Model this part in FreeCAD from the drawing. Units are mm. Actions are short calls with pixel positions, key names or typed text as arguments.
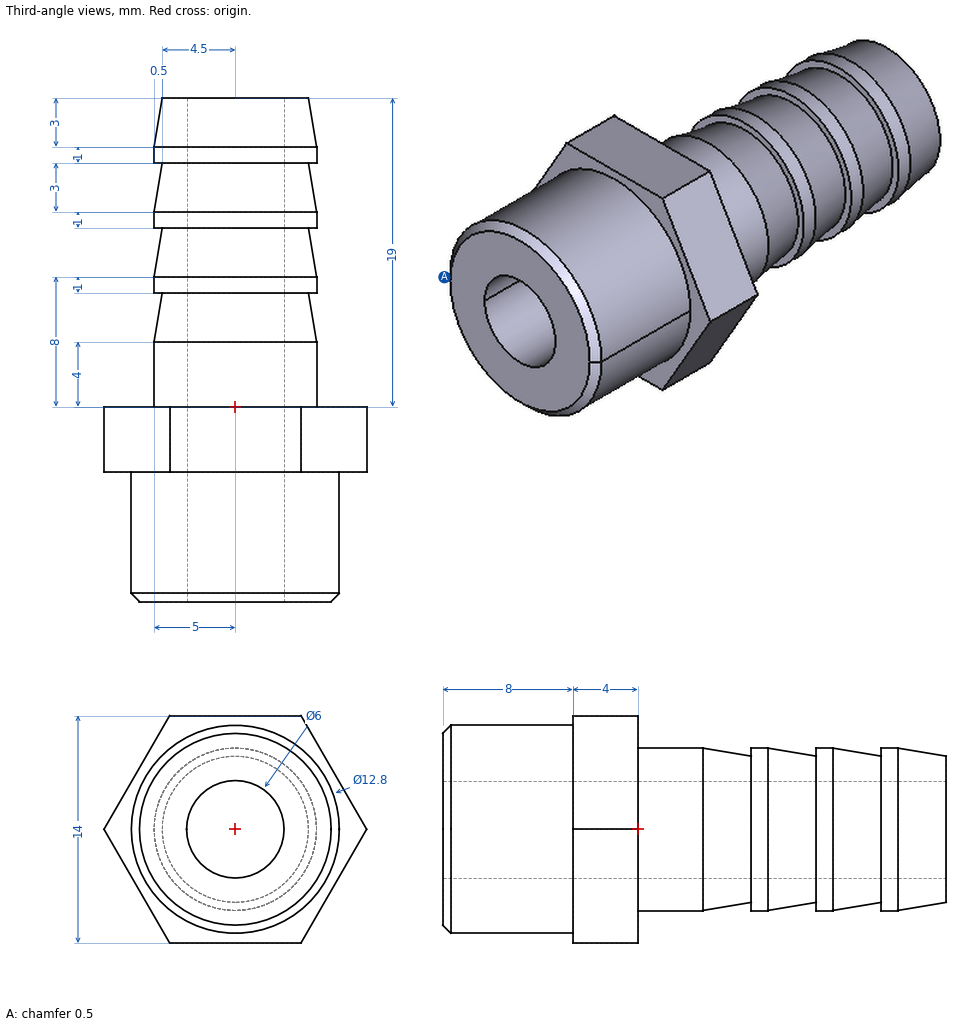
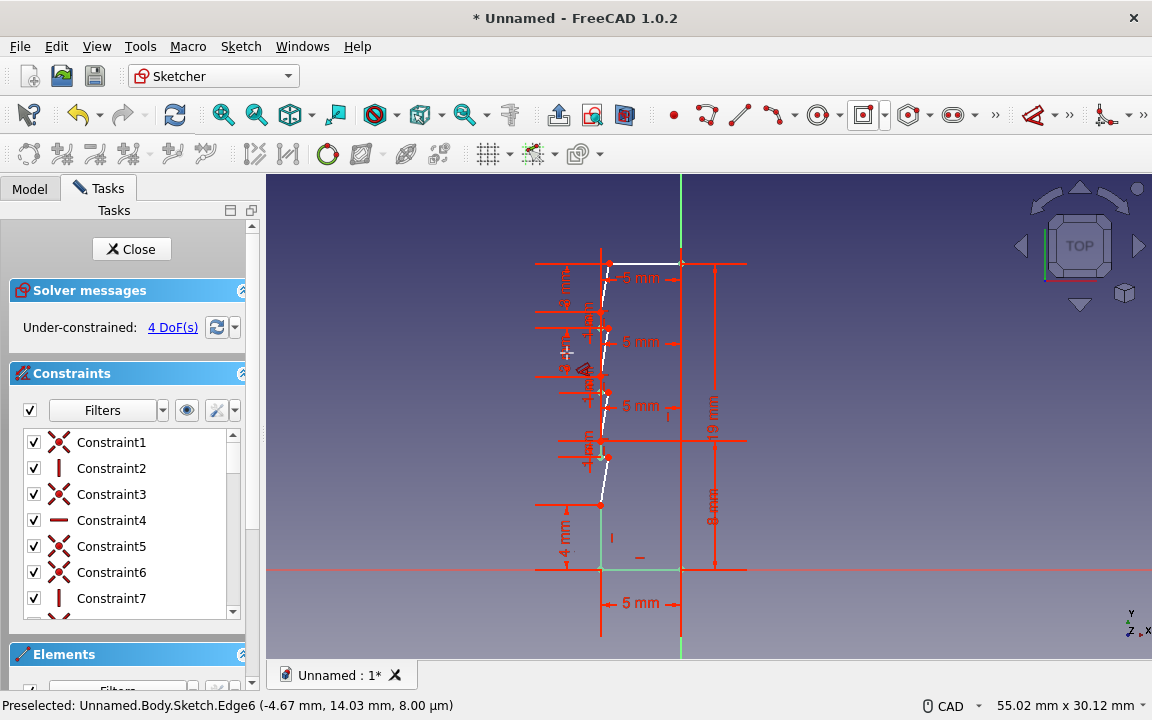
click(659, 264)
click(645, 230)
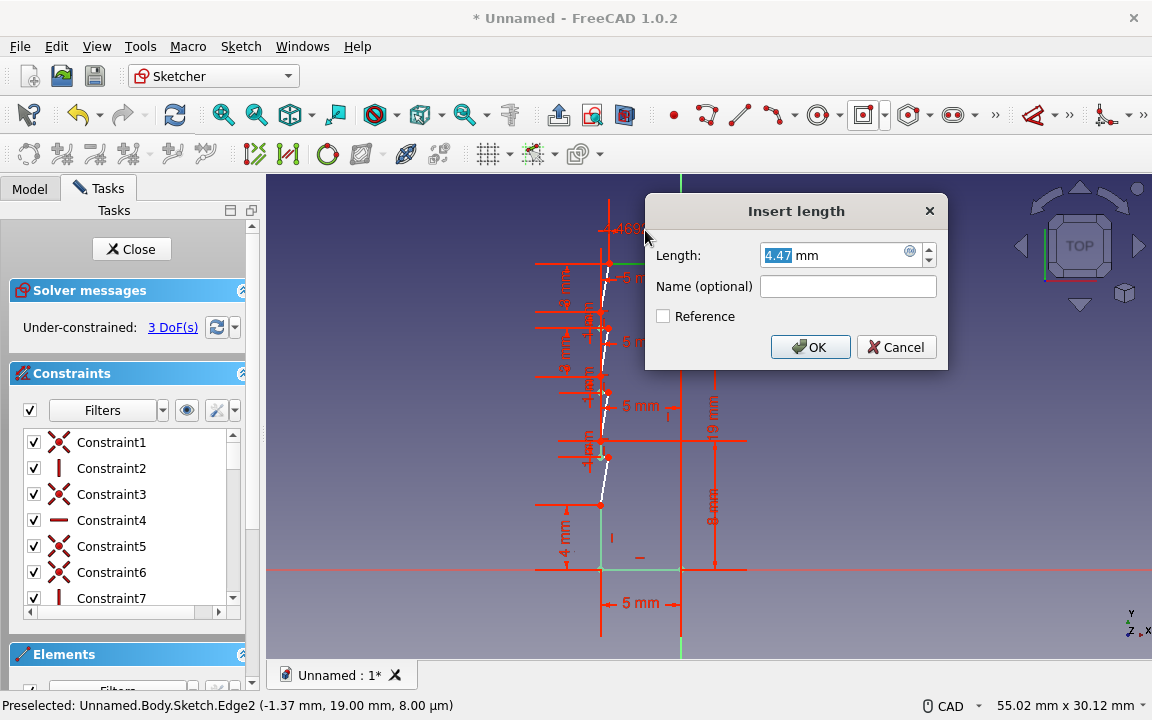
text(4.5)
key(Return)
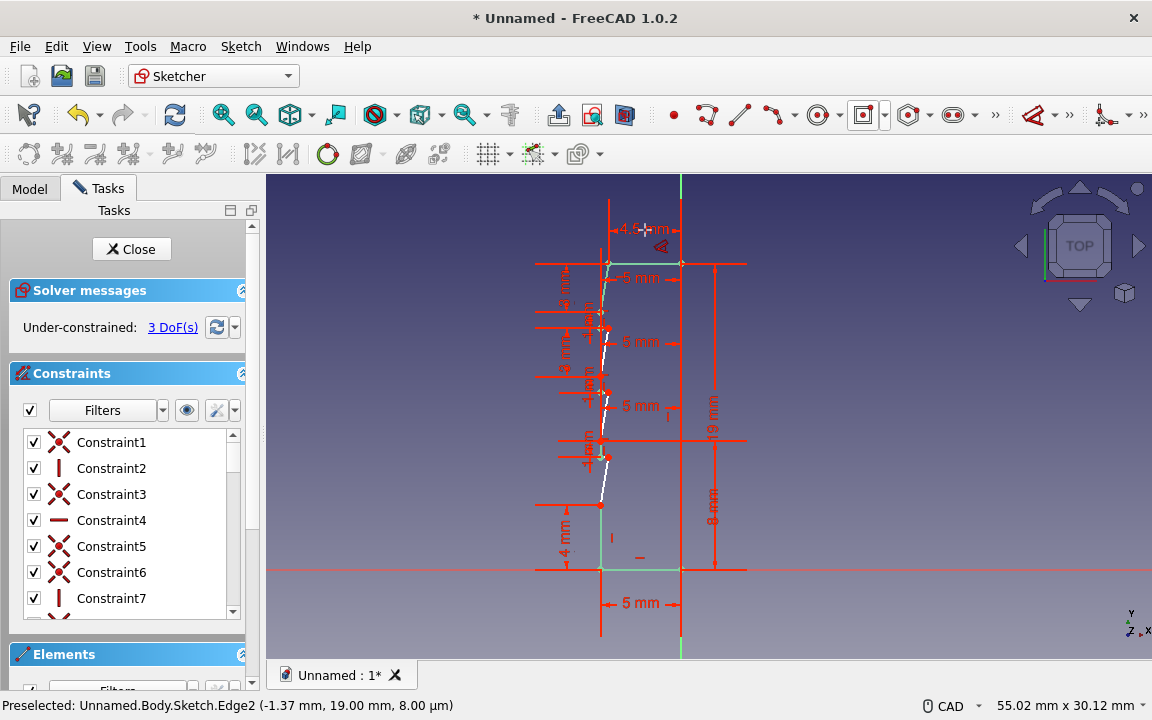
scroll(604, 328, up, 8)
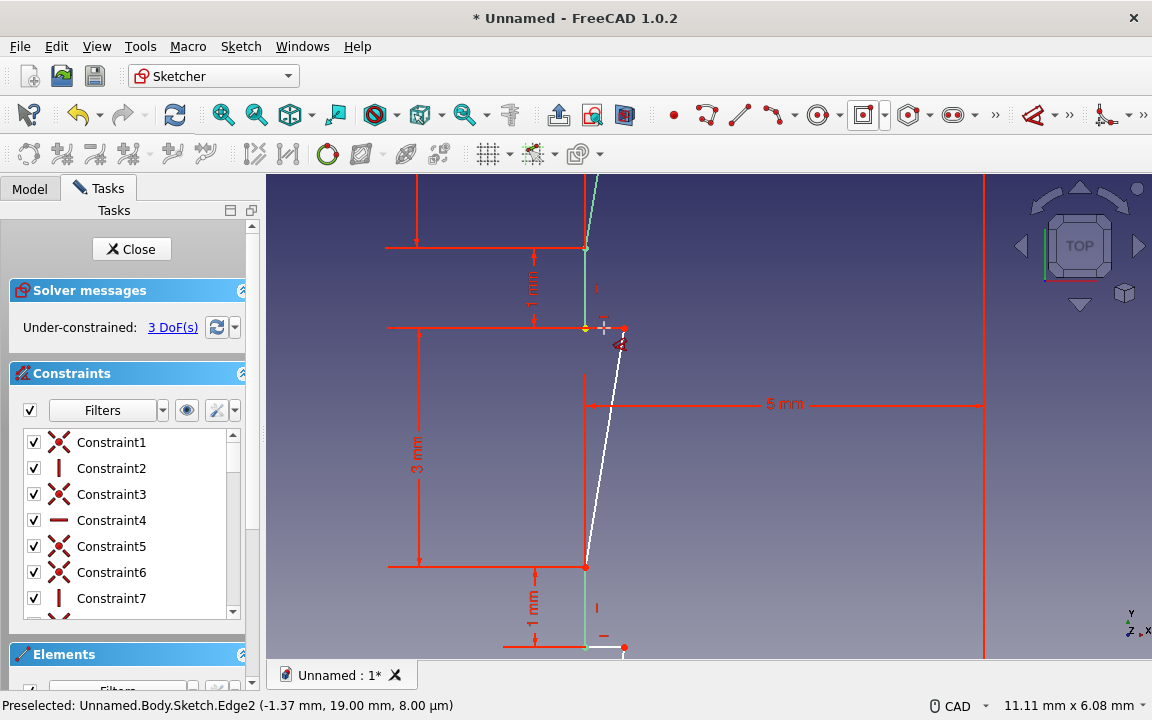
click(605, 328)
click(605, 294)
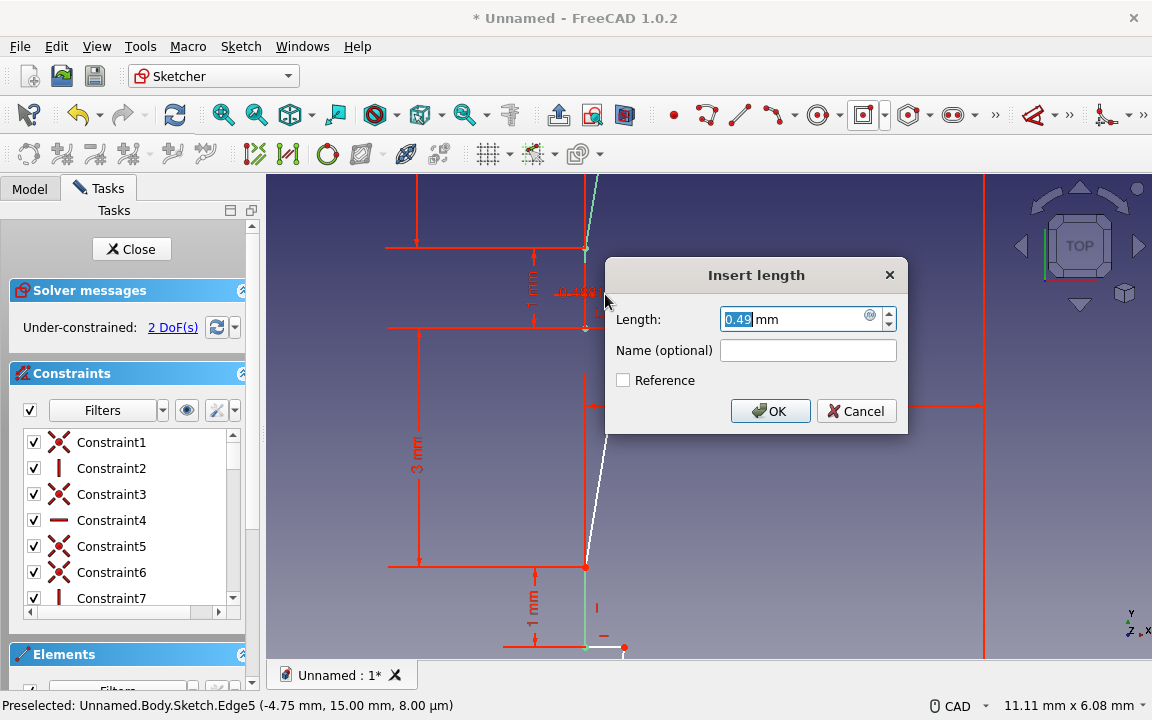
text(0.5)
key(Return)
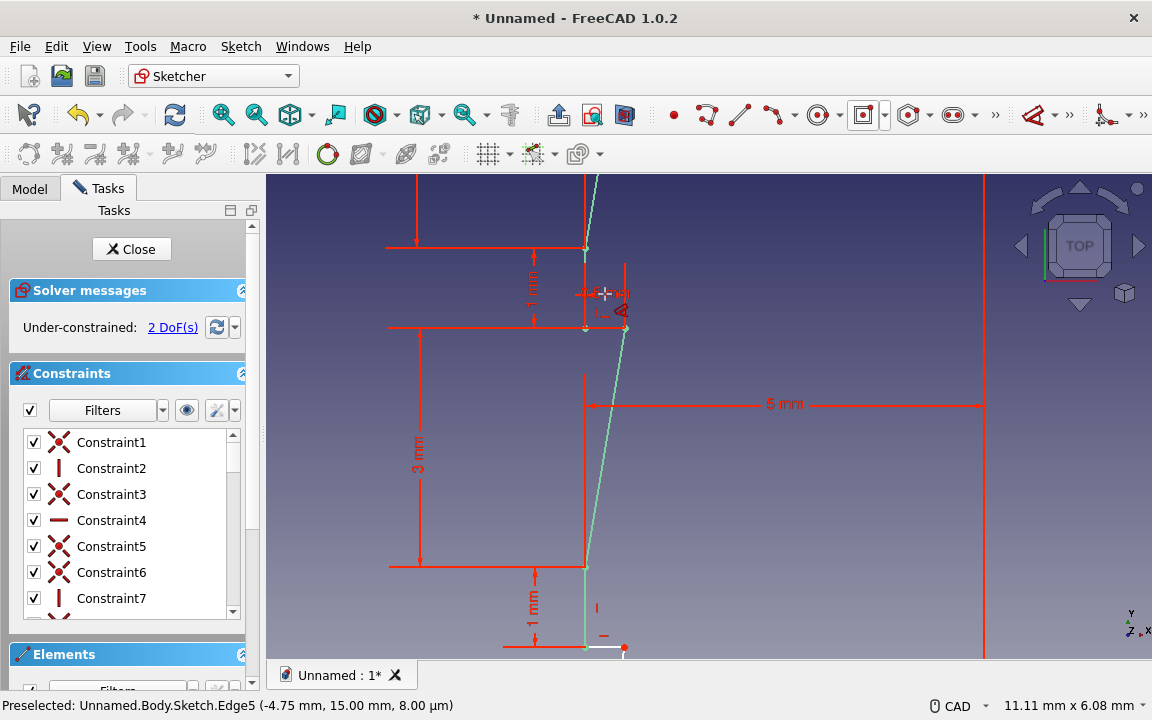
scroll(604, 328, down, 8)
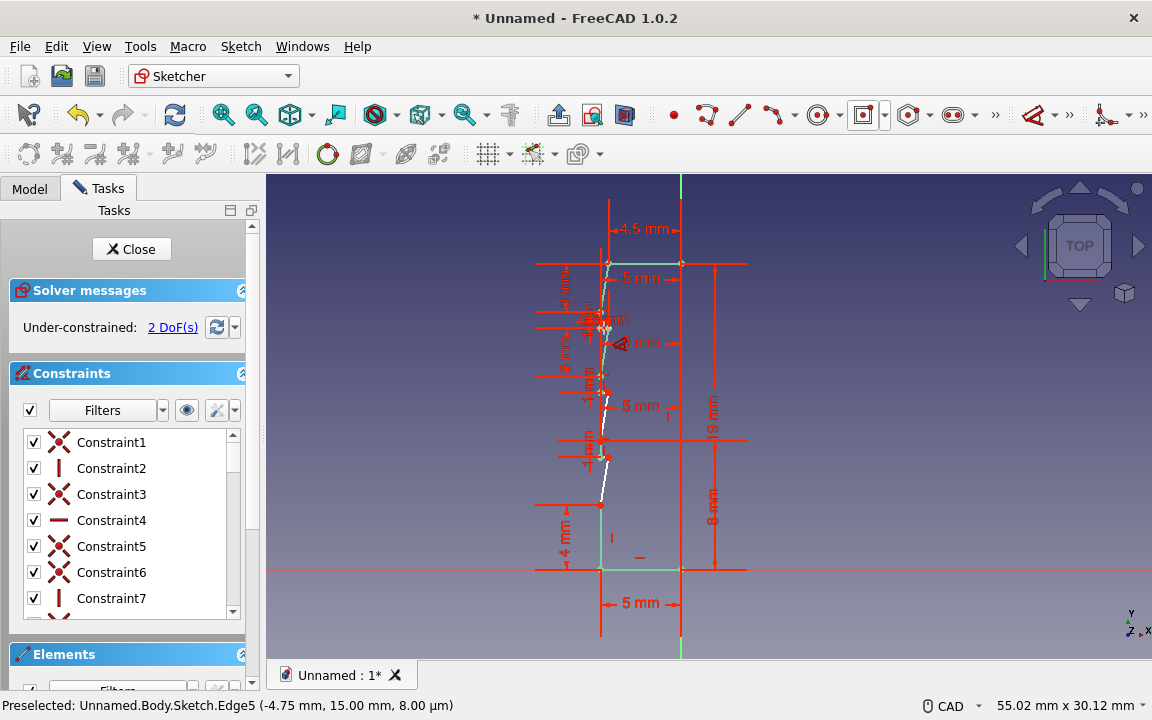
scroll(603, 393, up, 9)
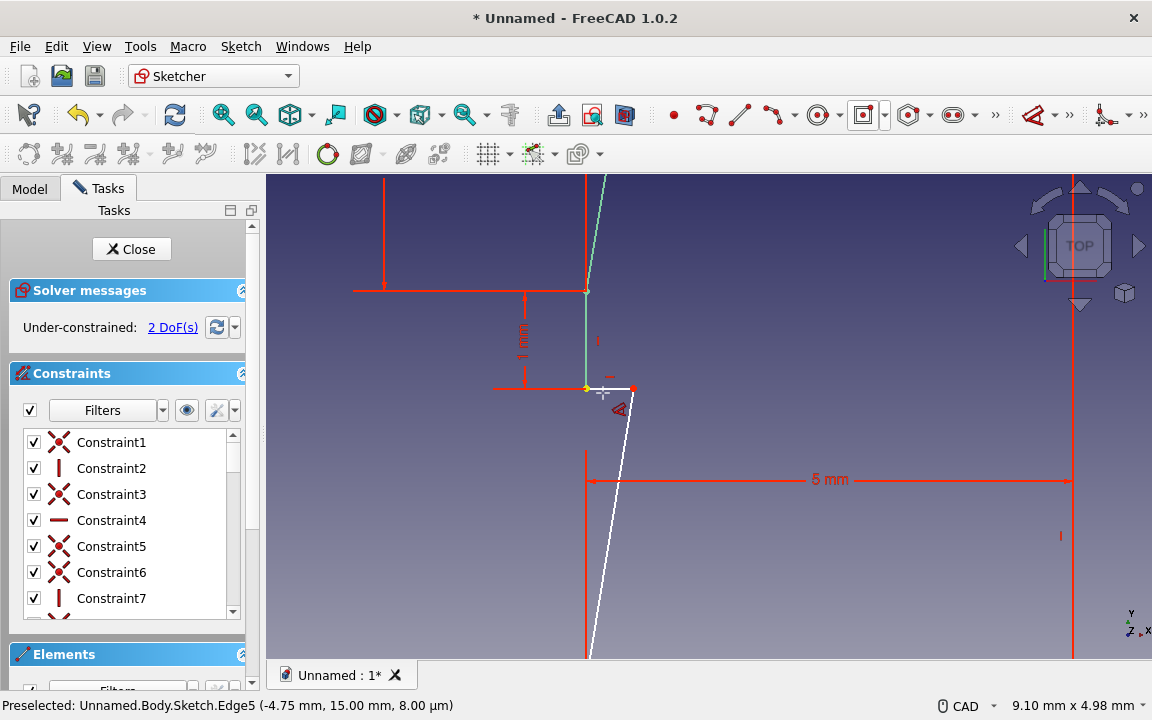
click(601, 389)
click(610, 355)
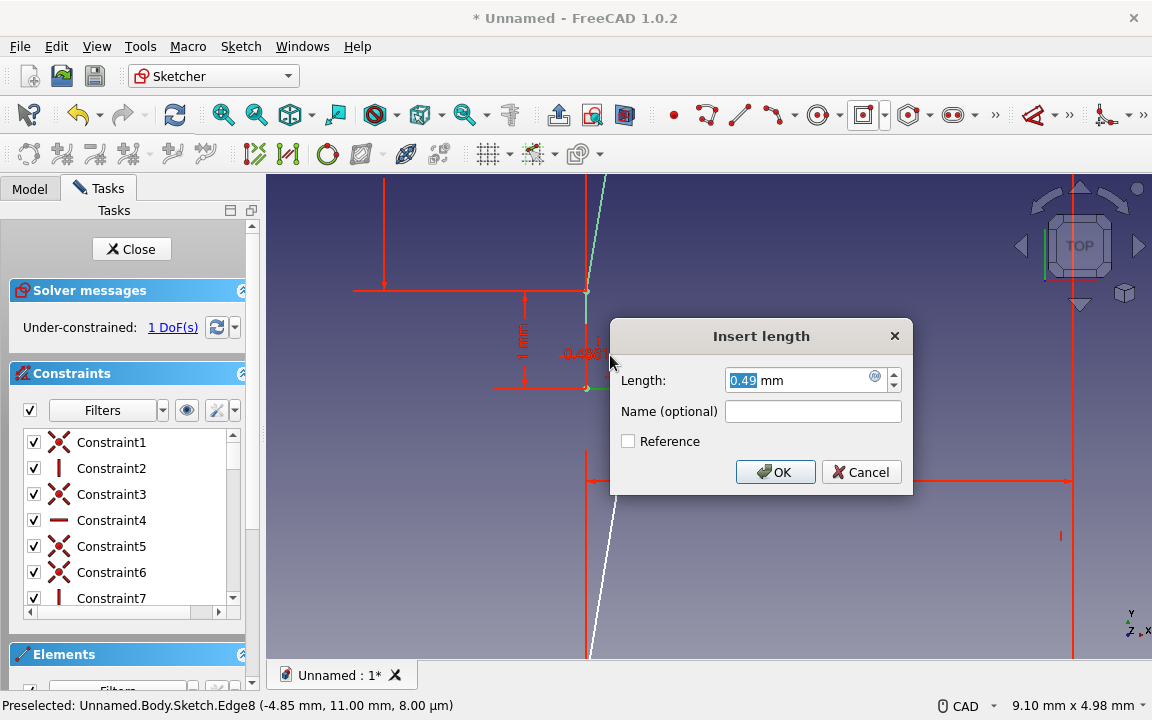
text(0.5)
key(Return)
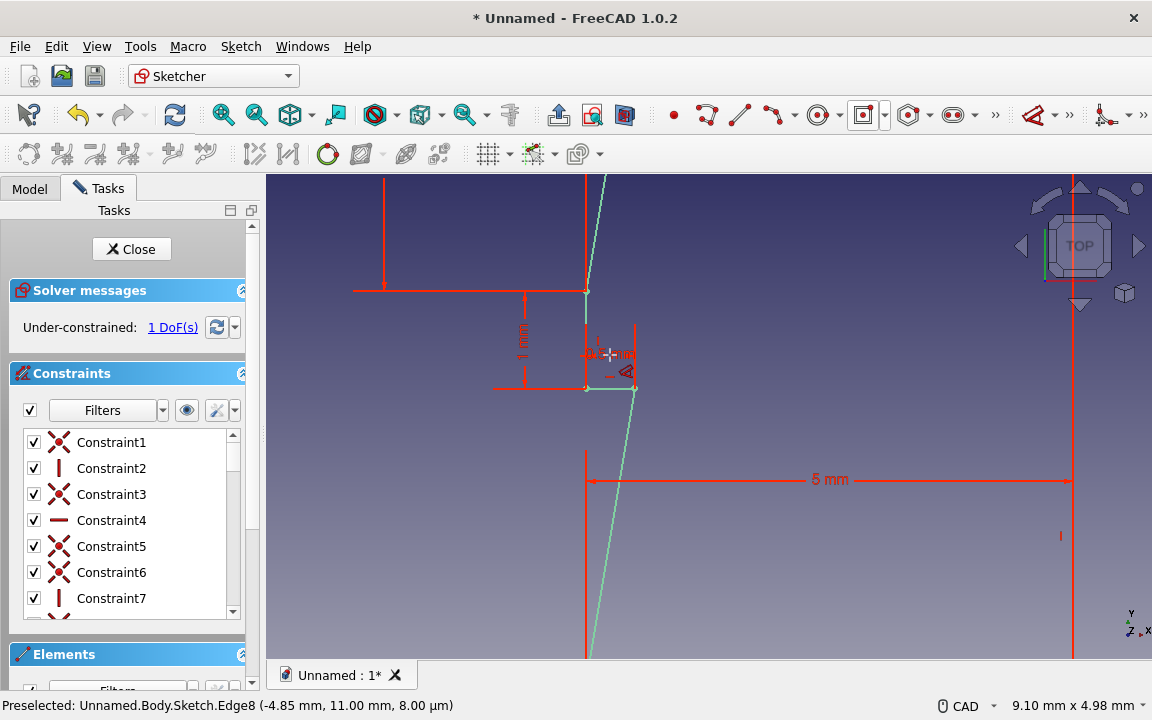
scroll(603, 393, down, 9)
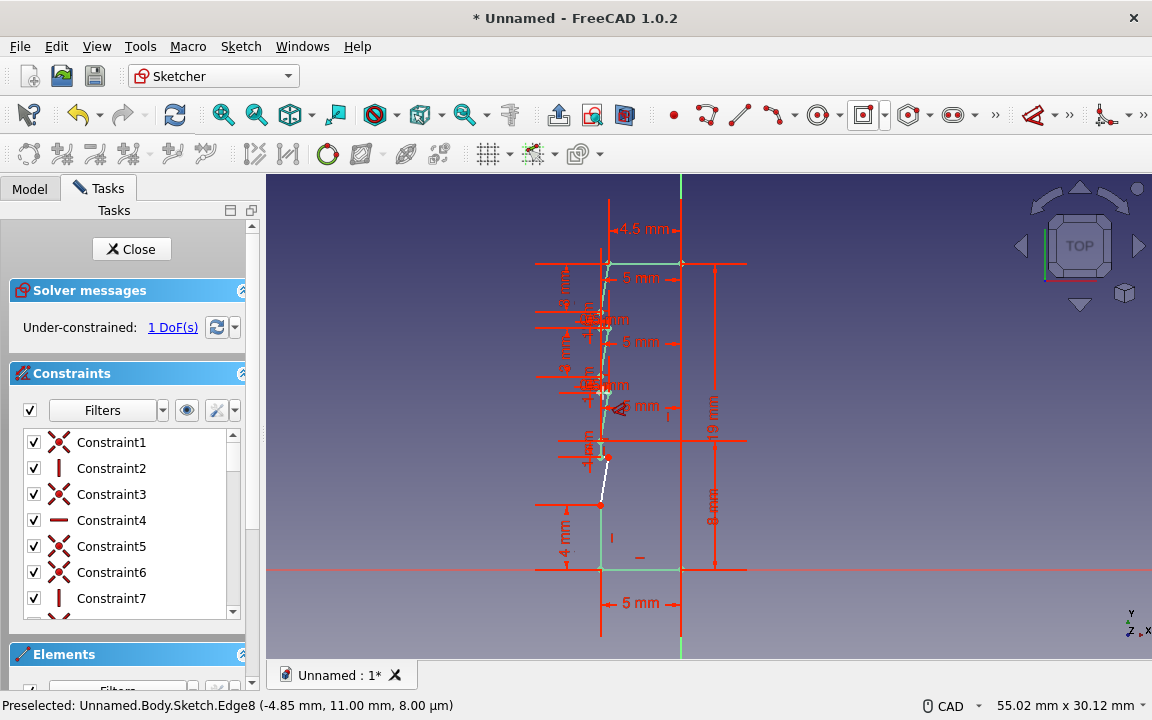
scroll(603, 457, up, 9)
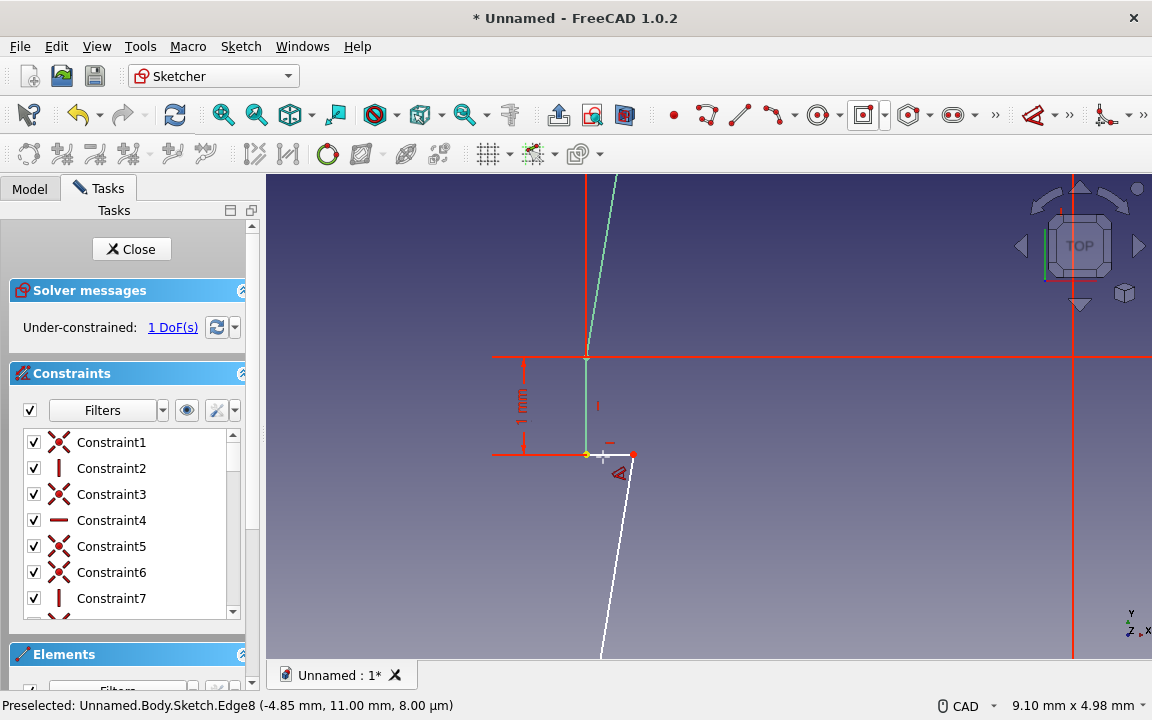
click(601, 455)
click(610, 489)